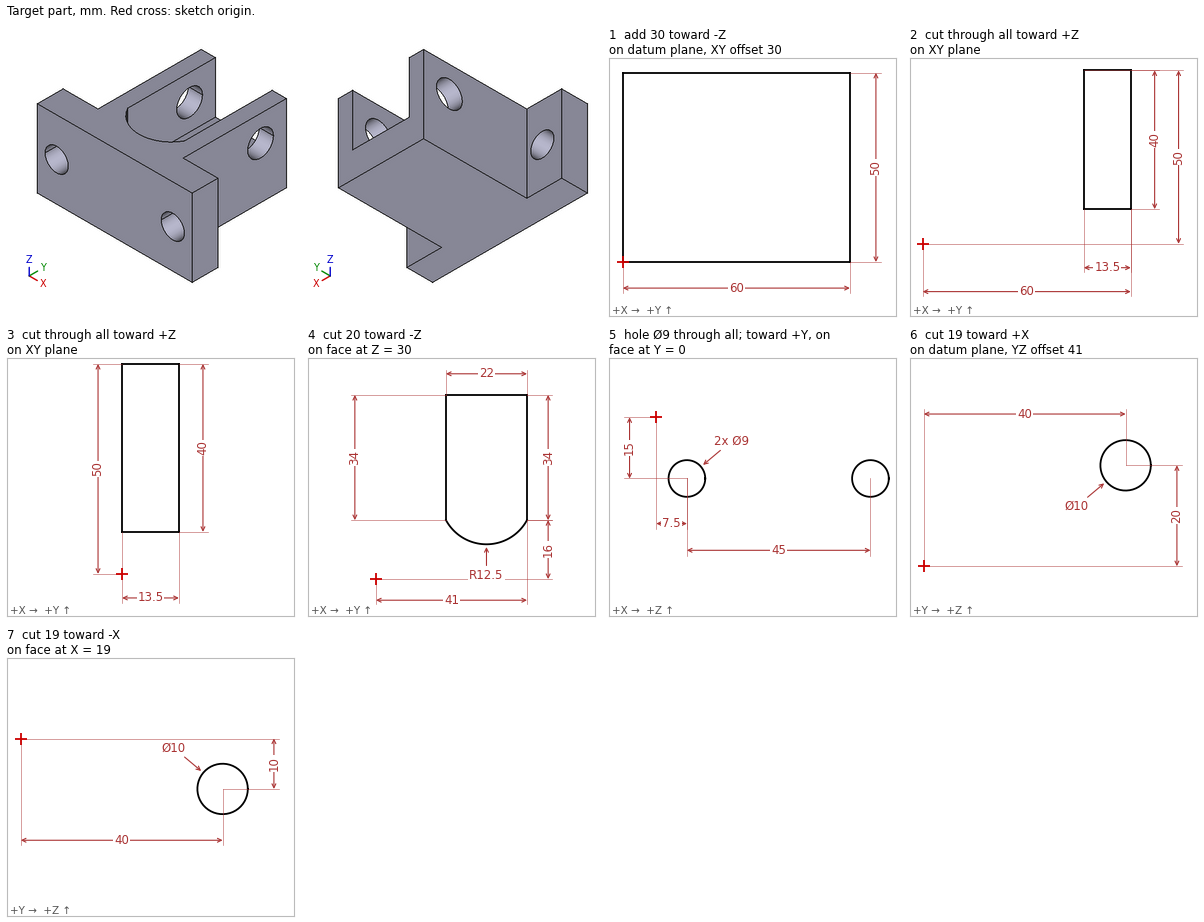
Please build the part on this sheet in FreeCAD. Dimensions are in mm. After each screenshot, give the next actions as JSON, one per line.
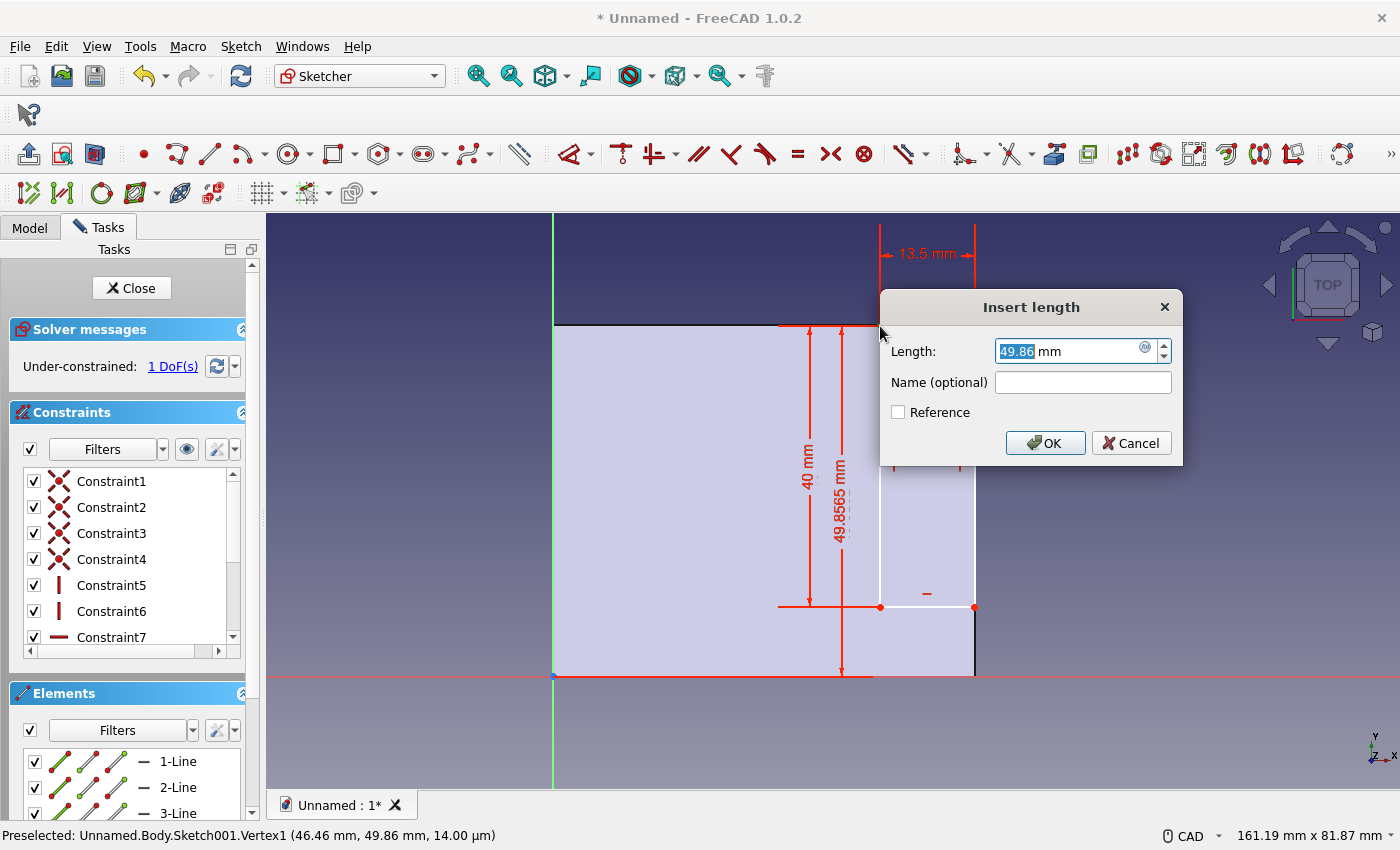
{"action": "type", "text": "50"}
{"action": "key", "text": "Return"}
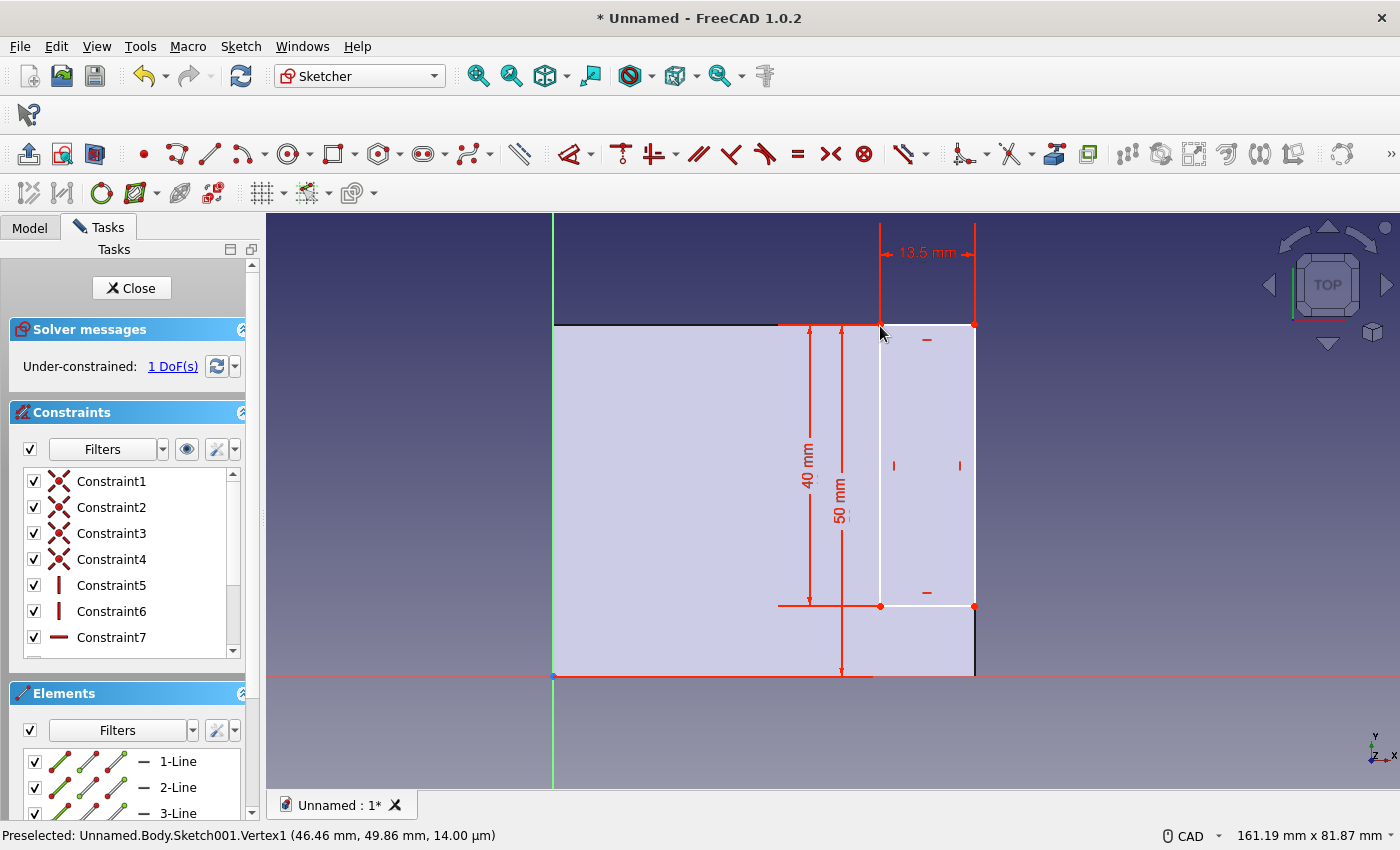
{"action": "left_click", "coordinate": [975, 606]}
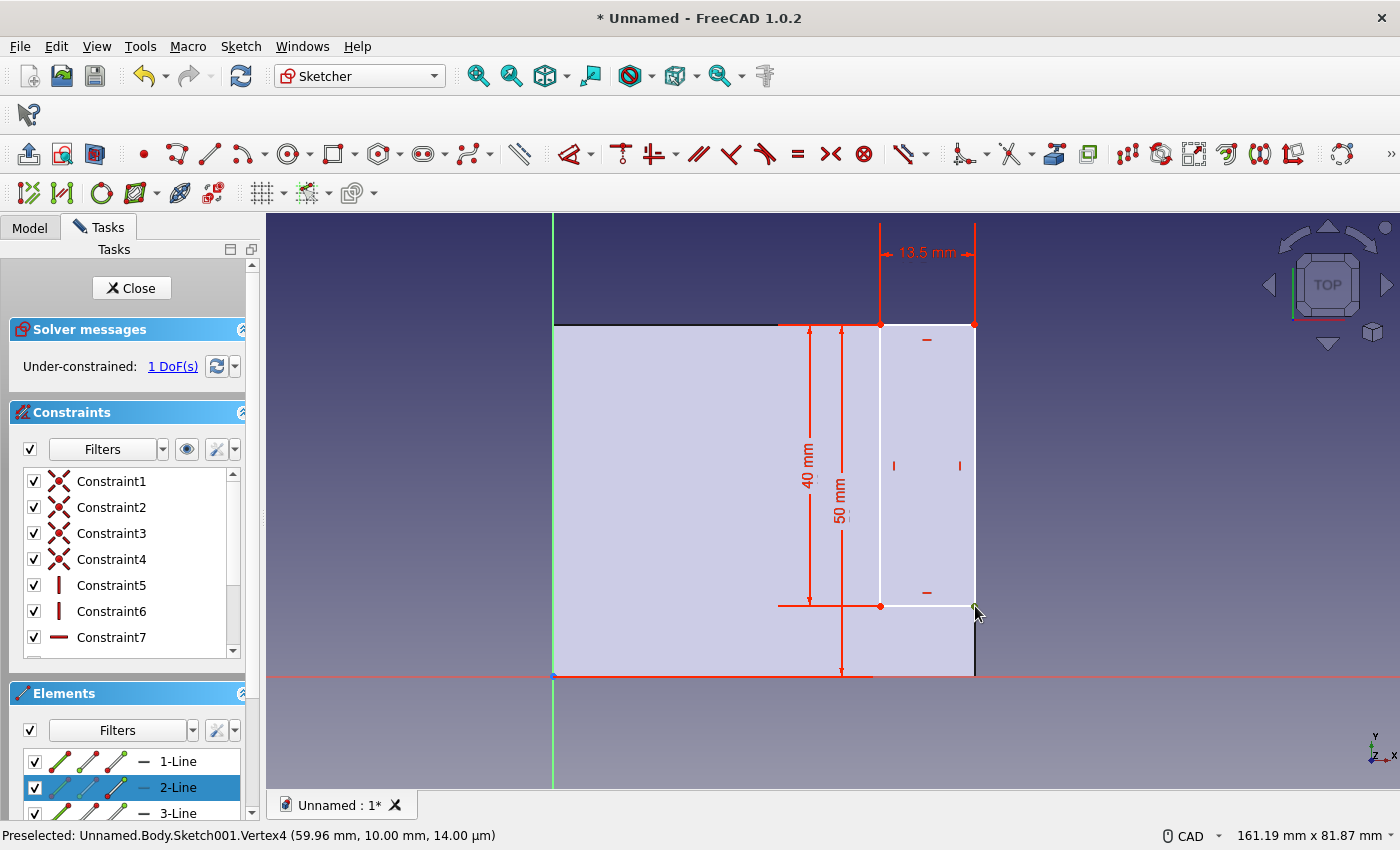
{"action": "key", "text": "l"}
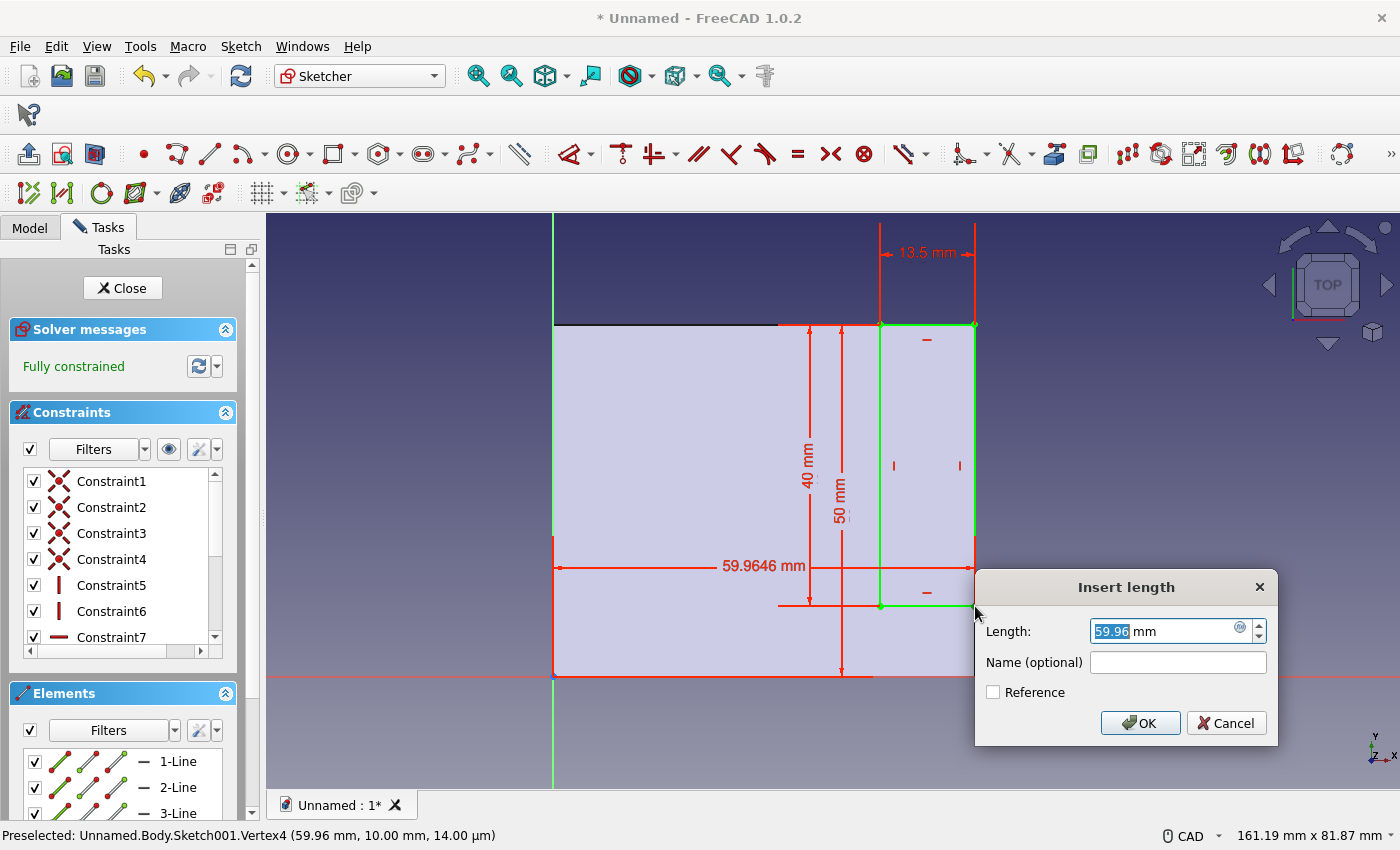
{"action": "type", "text": "60"}
{"action": "key", "text": "Return"}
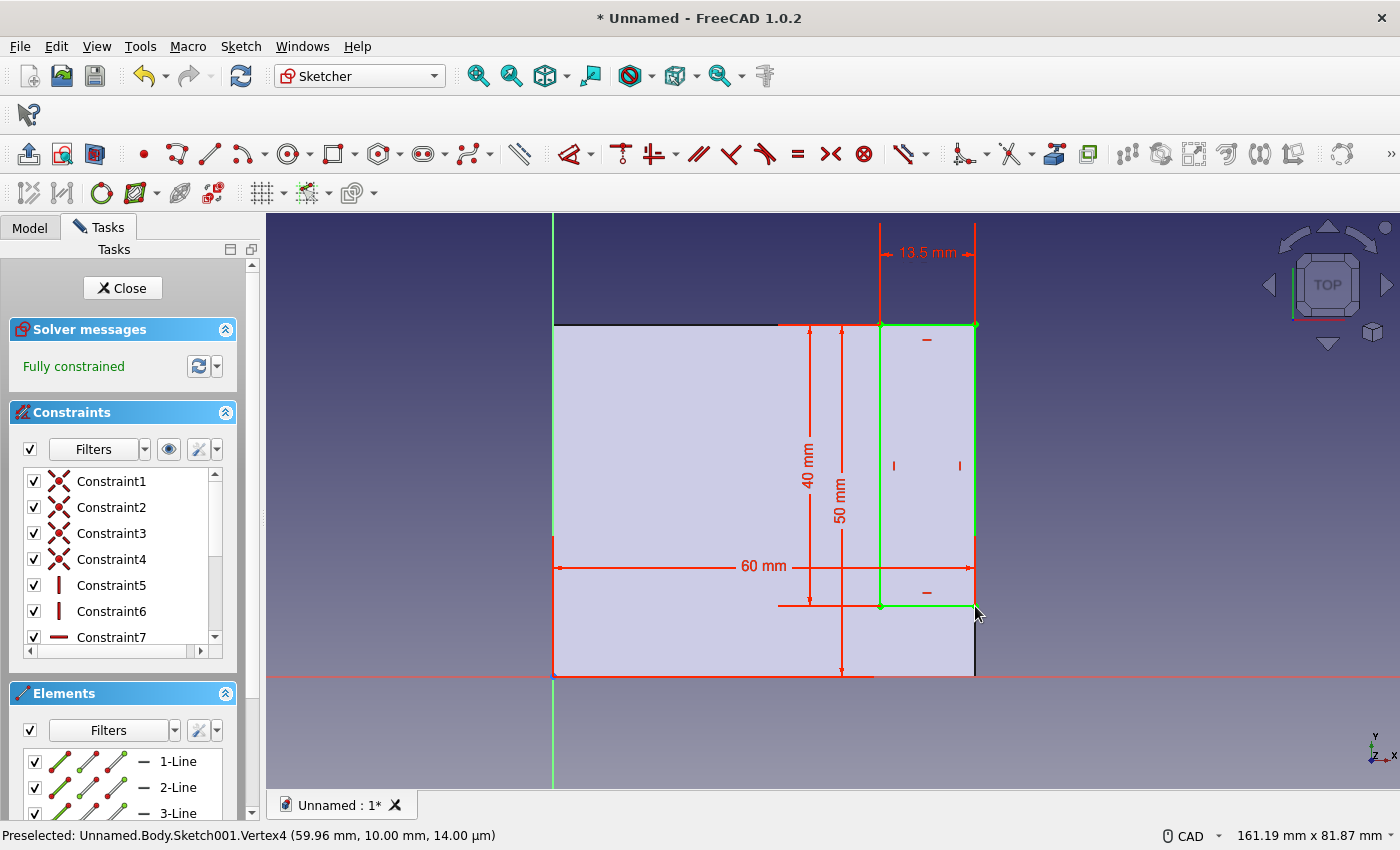
{"action": "left_click", "coordinate": [123, 288]}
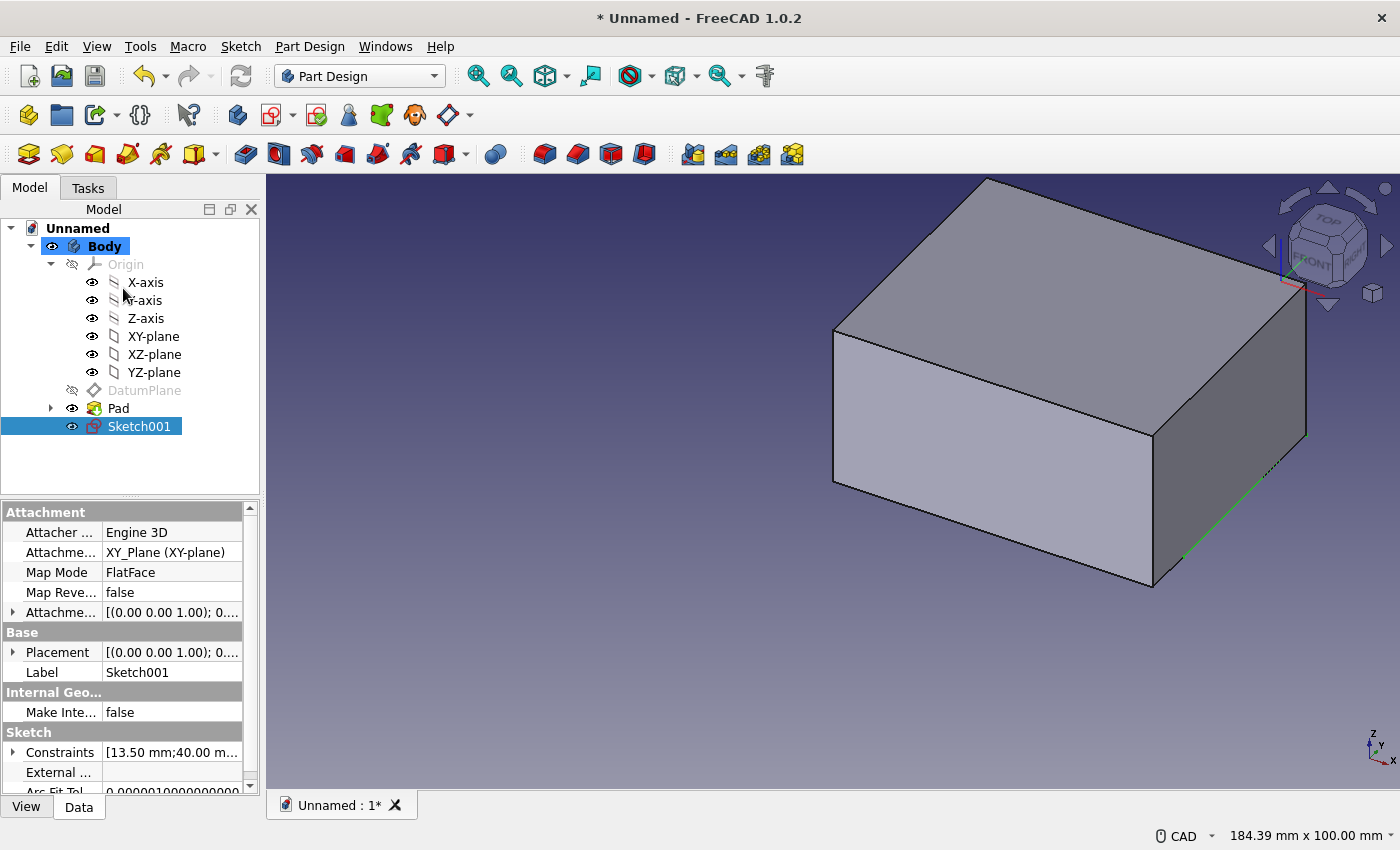
{"action": "left_click", "coordinate": [246, 154]}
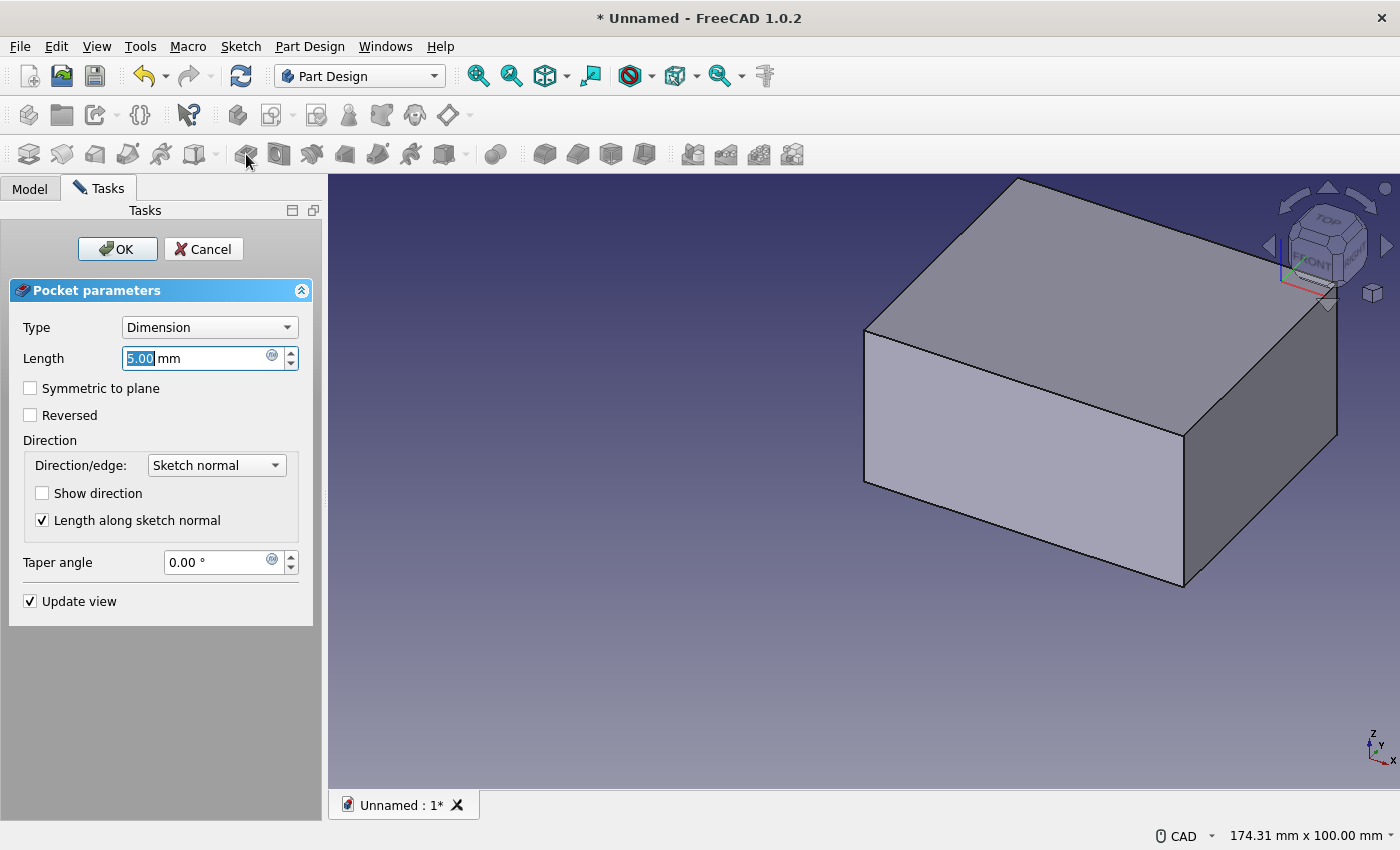
{"action": "left_click", "coordinate": [210, 328]}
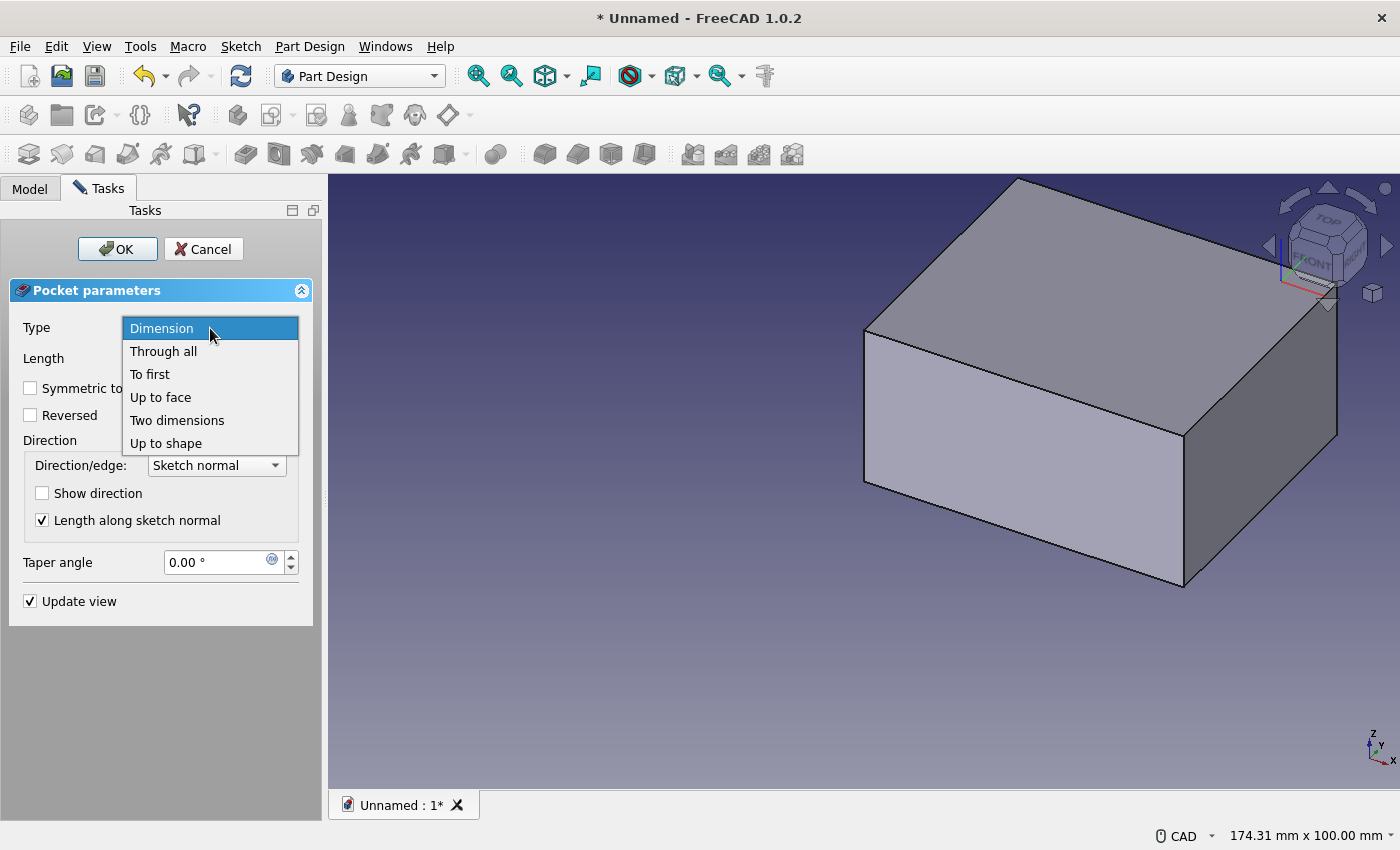
{"action": "left_click", "coordinate": [208, 352]}